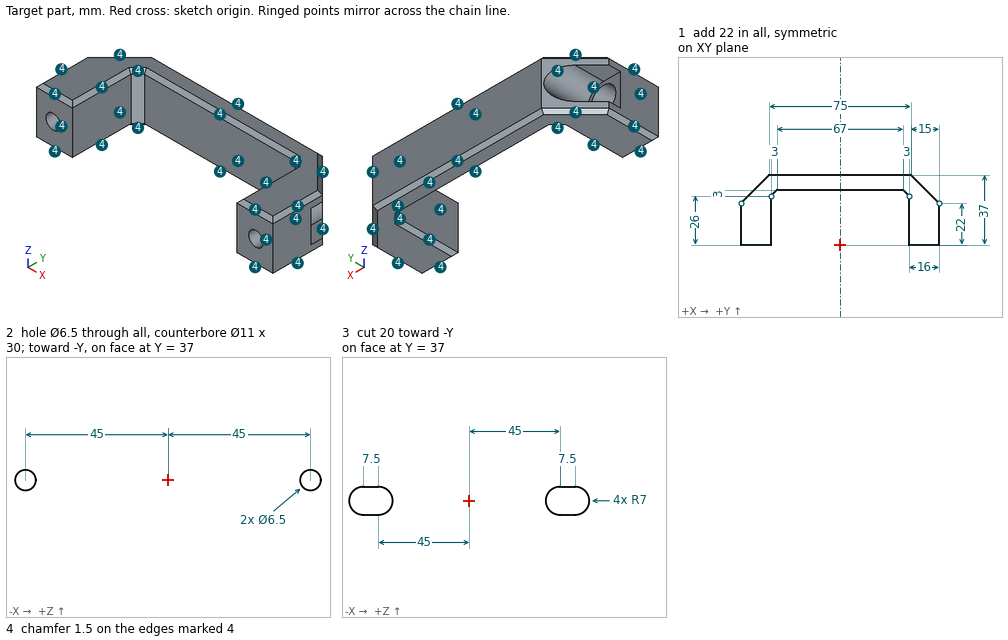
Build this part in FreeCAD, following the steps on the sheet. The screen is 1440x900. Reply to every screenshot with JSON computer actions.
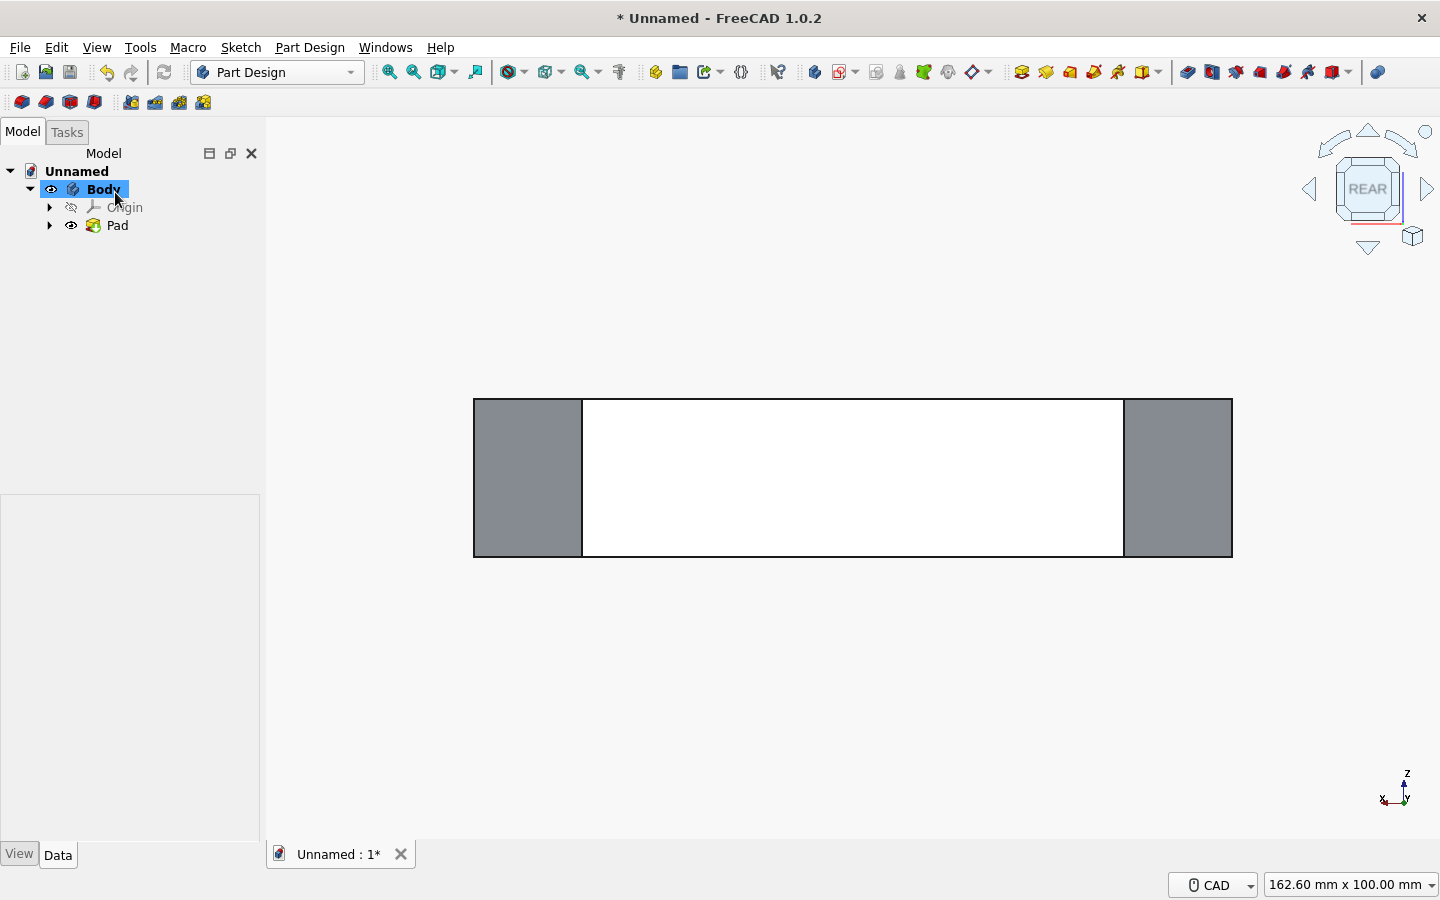
{"action": "left_click", "coordinate": [698, 477]}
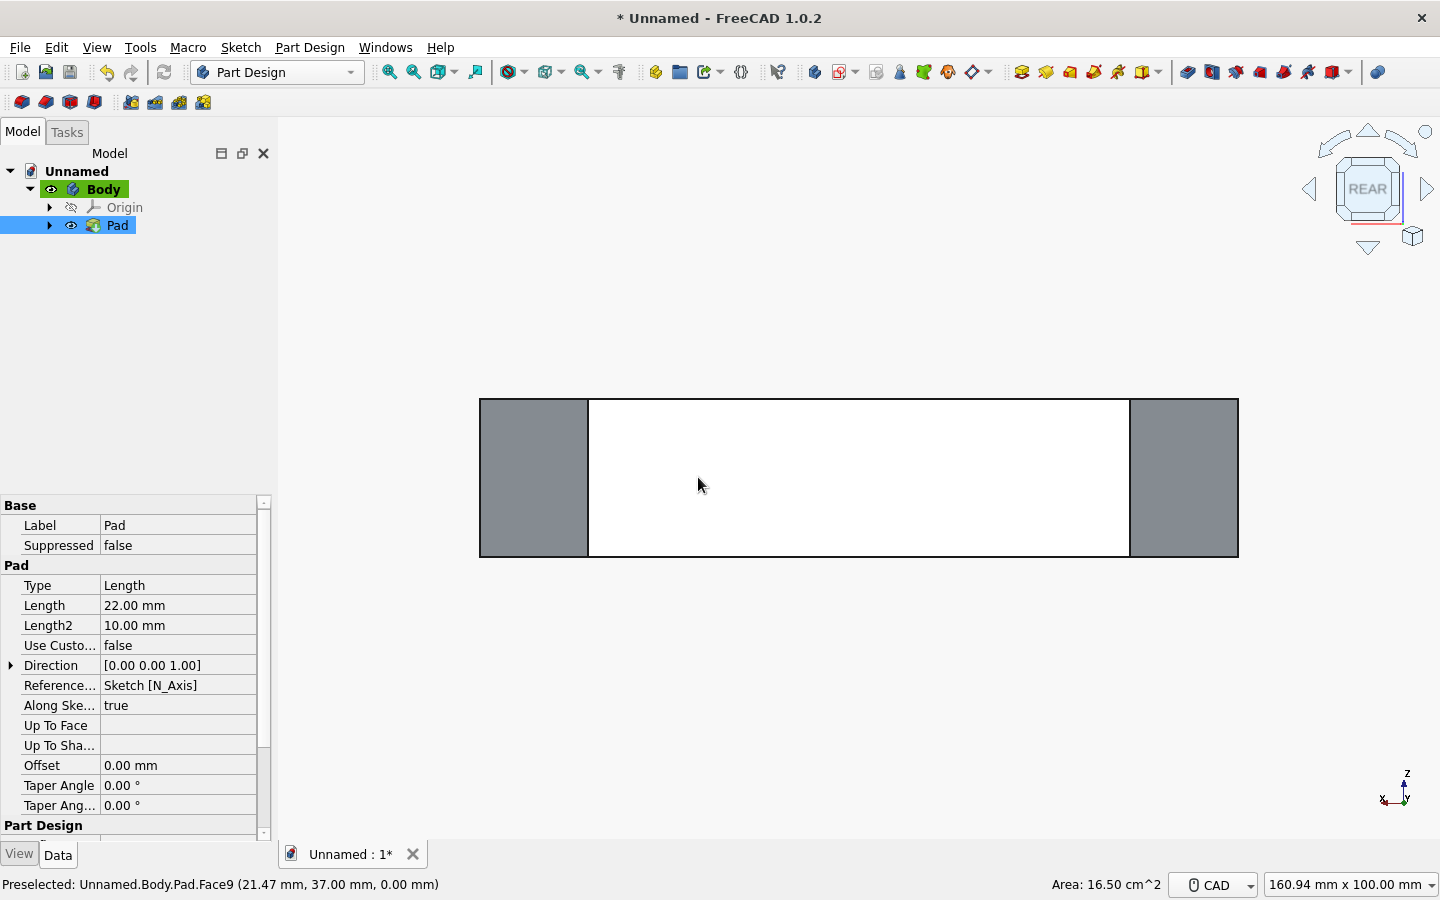
{"action": "left_click", "coordinate": [840, 72]}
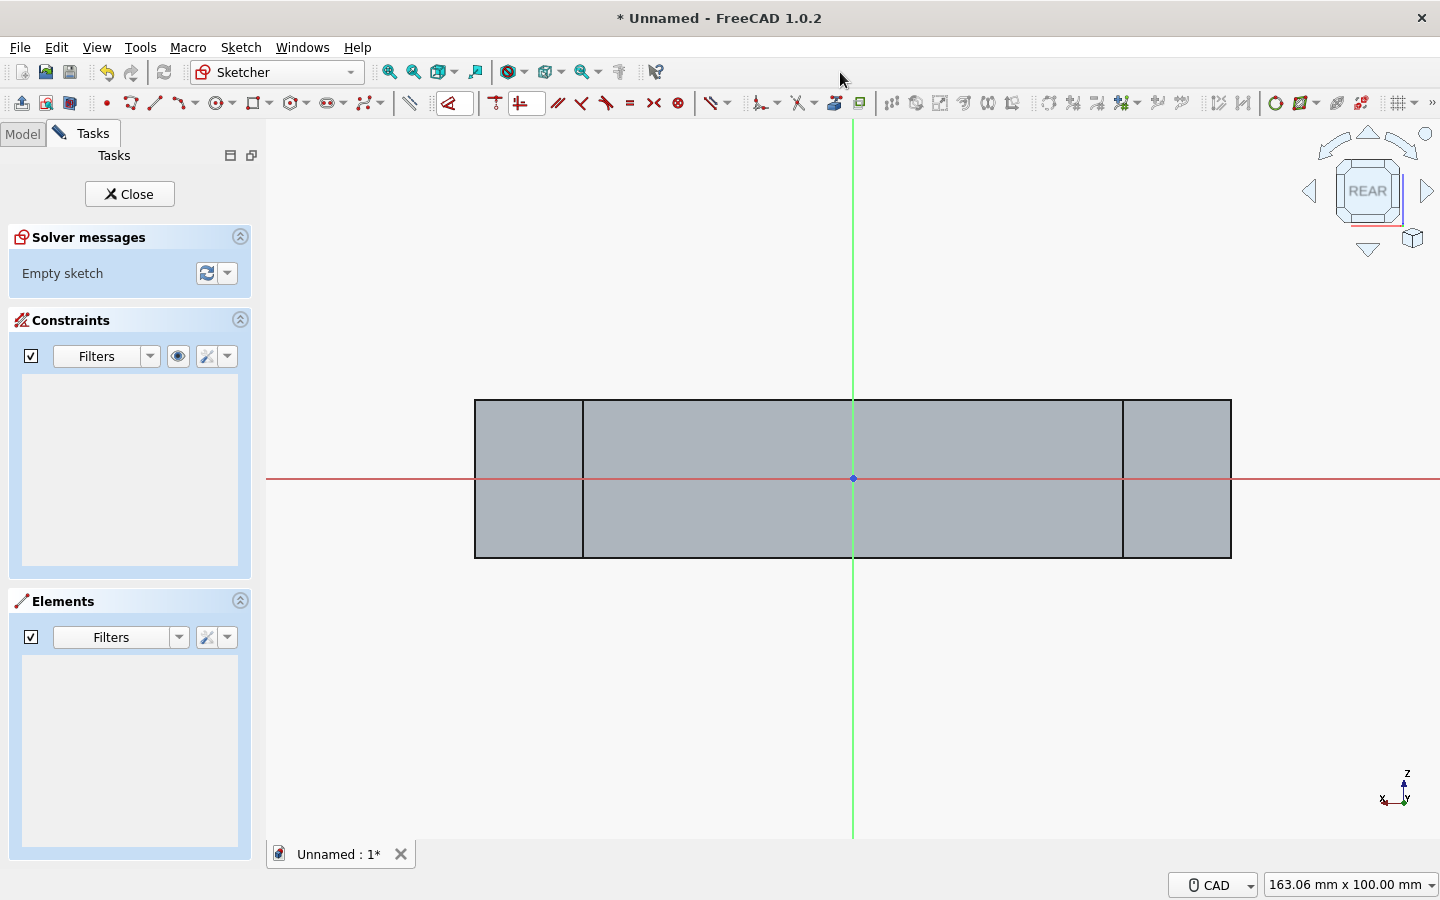
{"action": "left_click", "coordinate": [216, 104]}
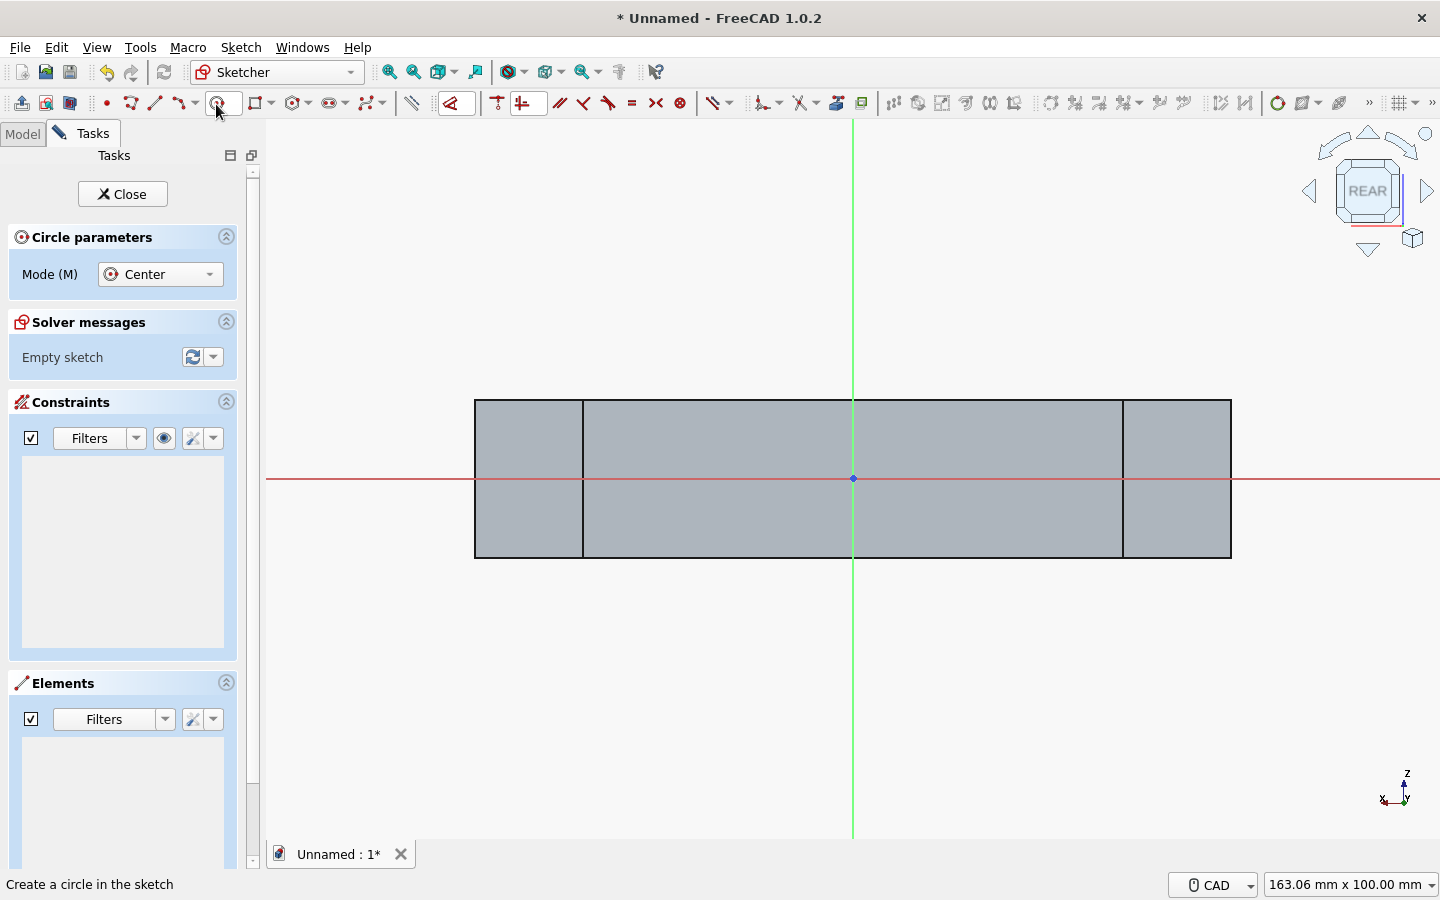
{"action": "left_click", "coordinate": [1177, 479]}
{"action": "left_click", "coordinate": [1194, 462]}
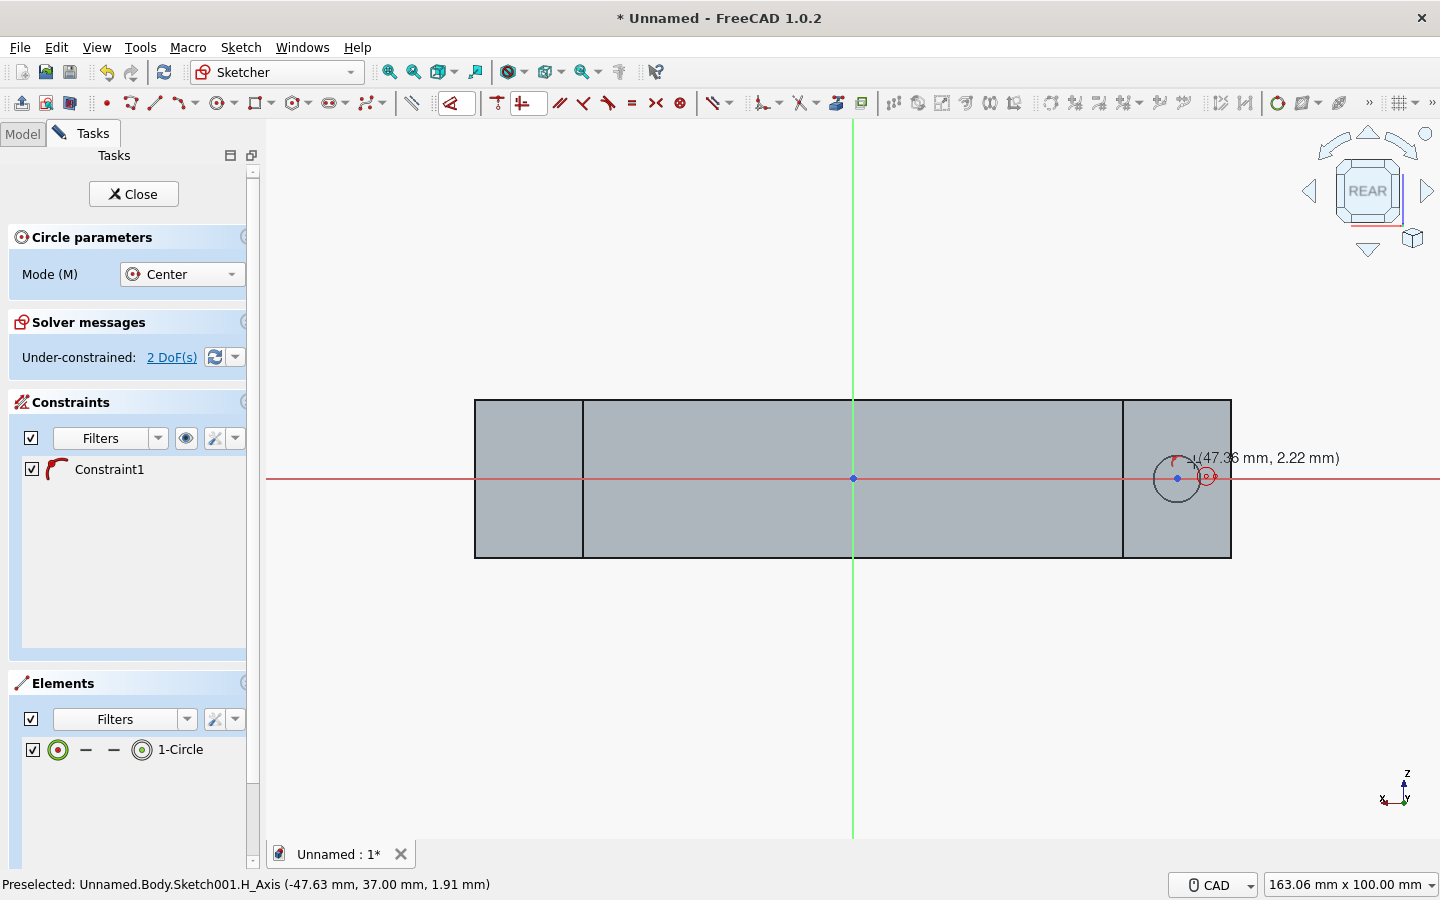
{"action": "left_click", "coordinate": [529, 479]}
{"action": "left_click", "coordinate": [546, 462]}
{"action": "key", "text": "Escape"}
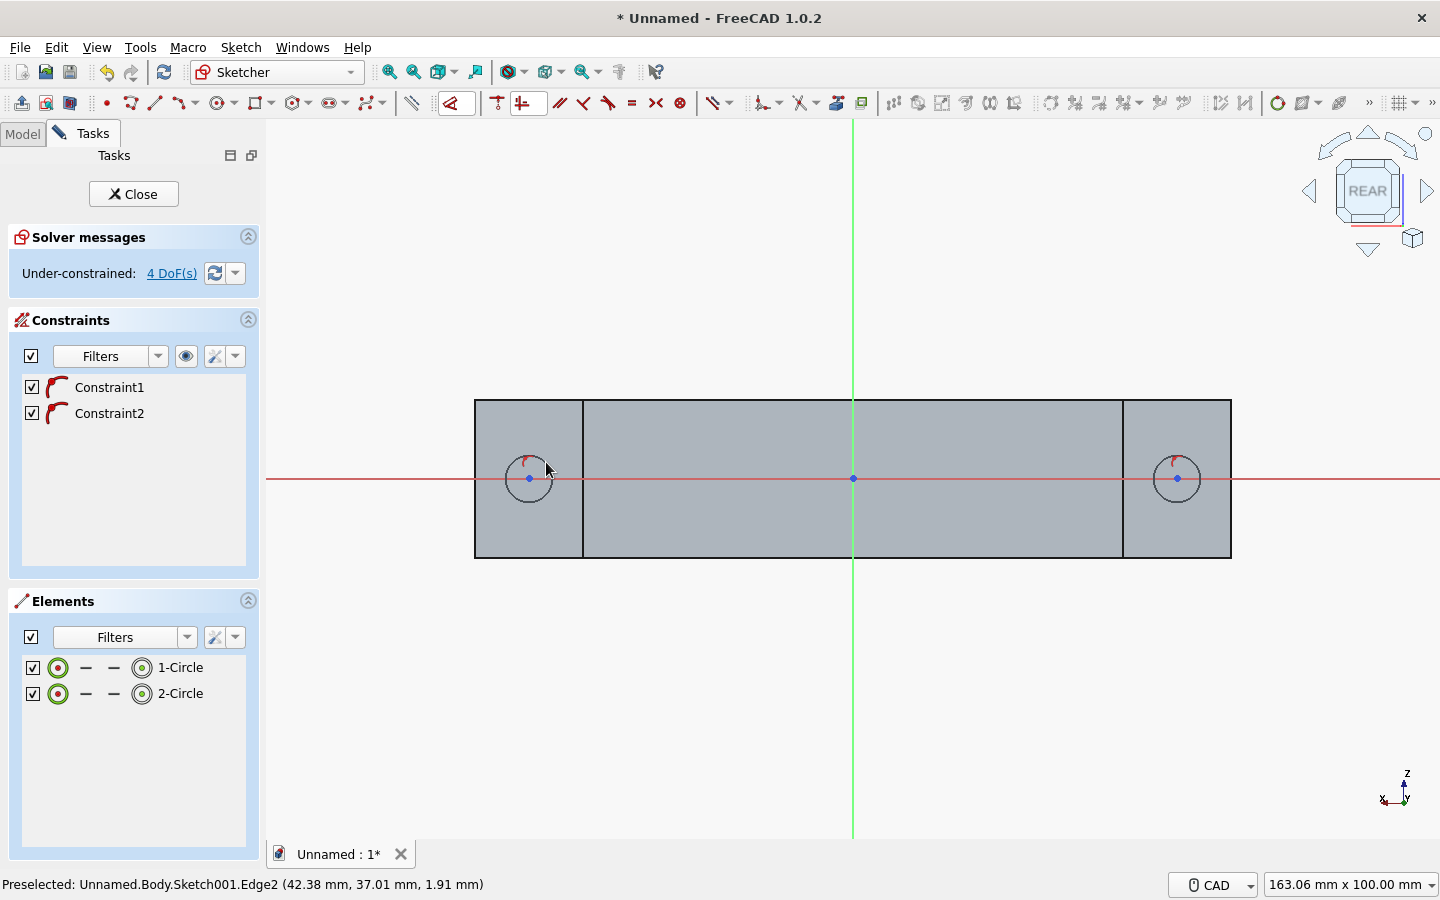
{"action": "left_click", "coordinate": [1193, 462]}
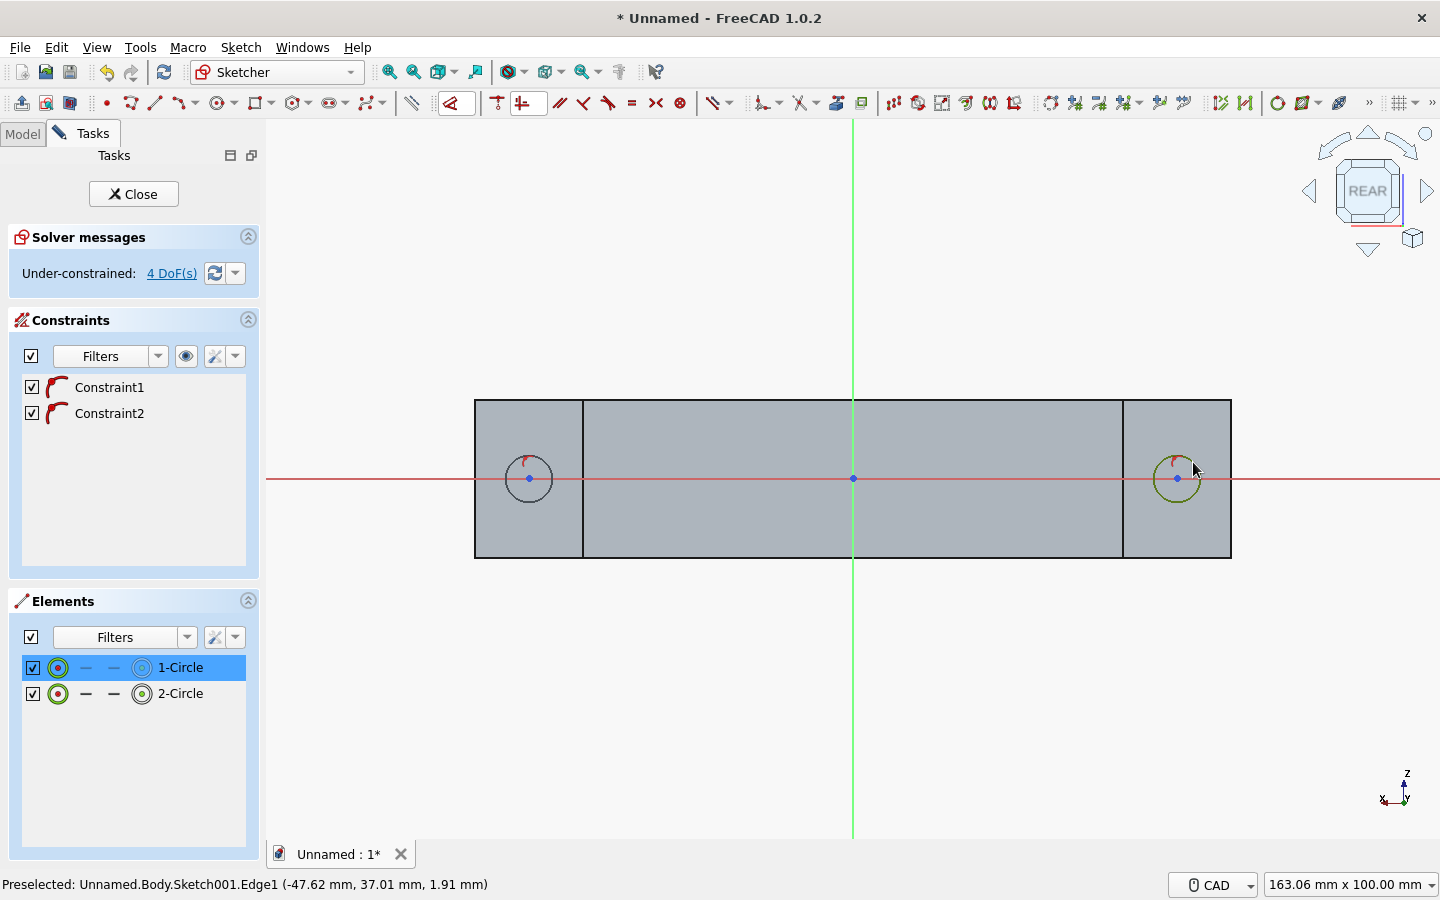
{"action": "left_click", "coordinate": [545, 462]}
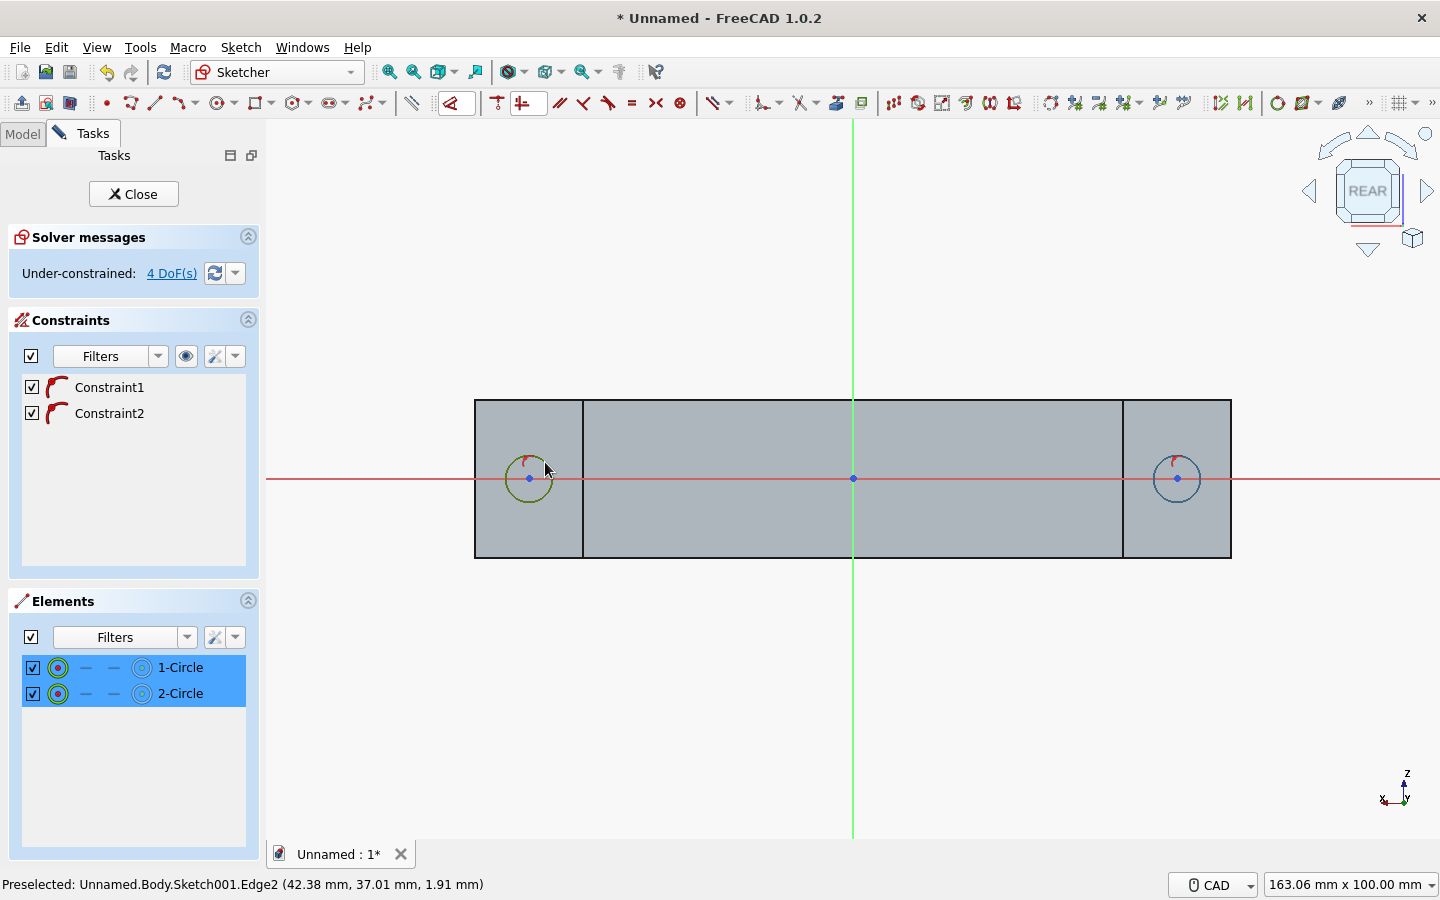
{"action": "left_click", "coordinate": [632, 104]}